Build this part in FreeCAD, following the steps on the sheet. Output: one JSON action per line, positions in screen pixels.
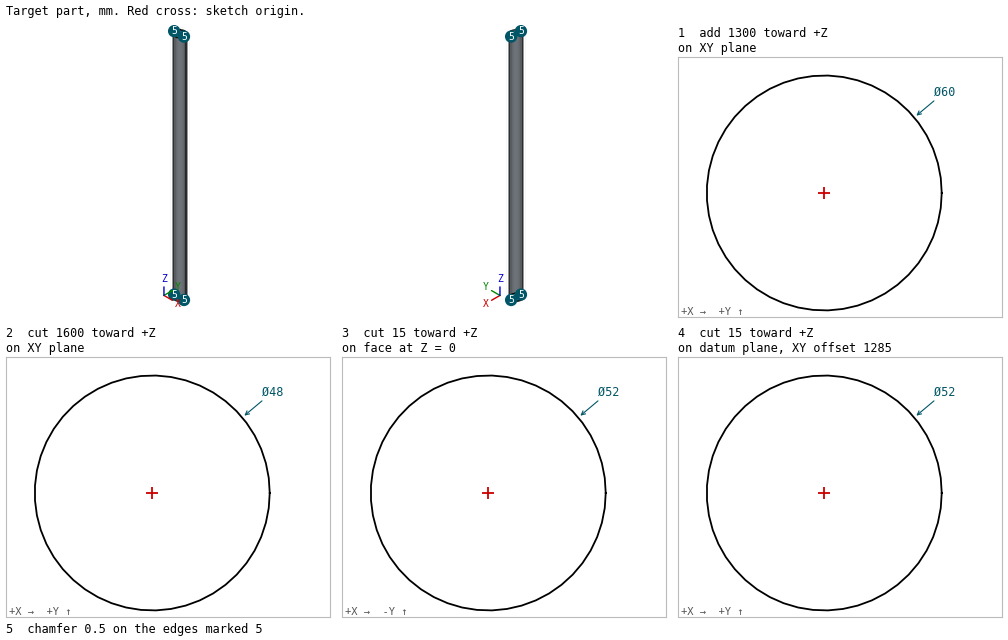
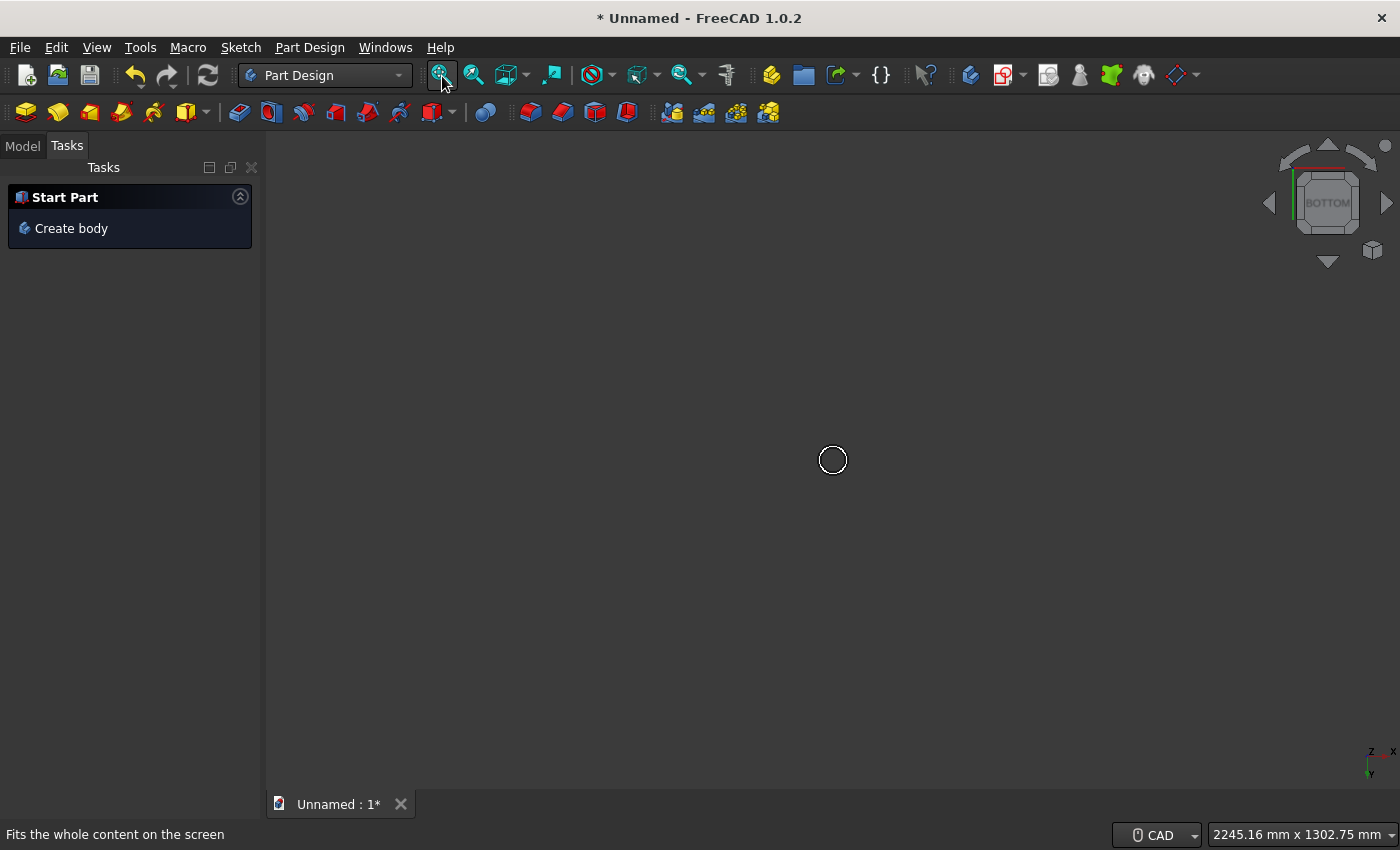
{"action": "scroll", "coordinate": [837, 472], "scroll_direction": "up", "scroll_amount": 11}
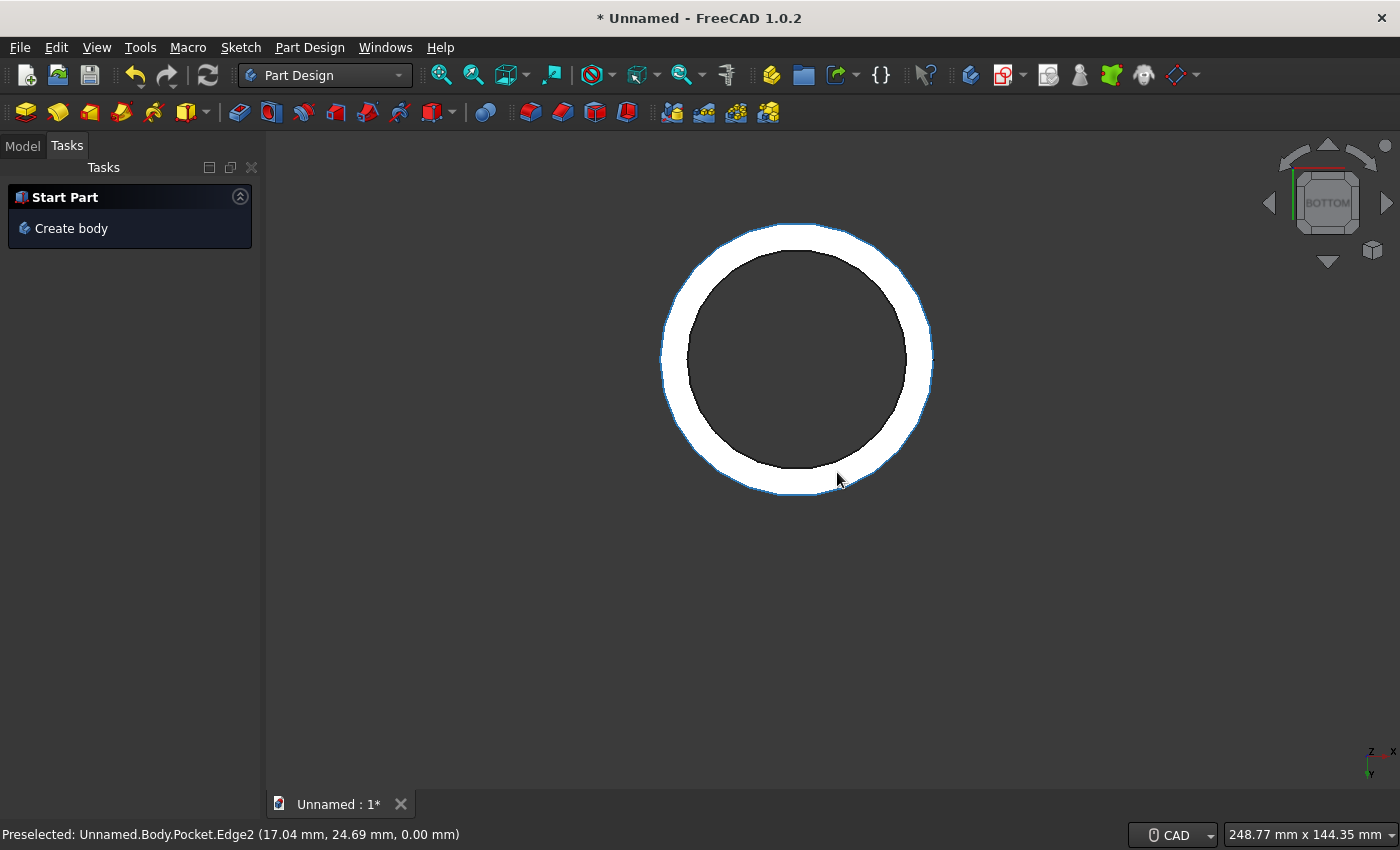
{"action": "left_click", "coordinate": [836, 476]}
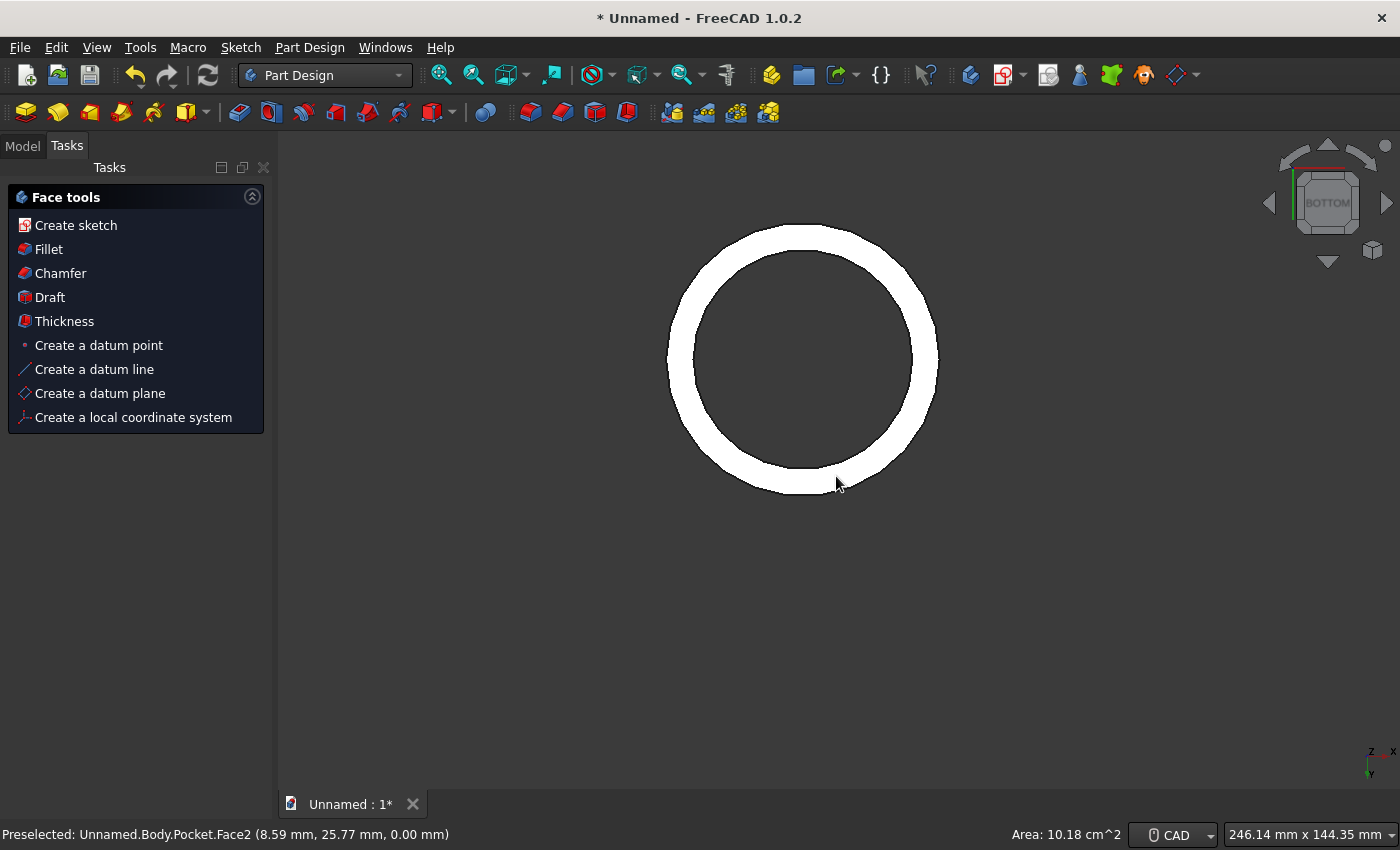
{"action": "left_click", "coordinate": [1004, 76]}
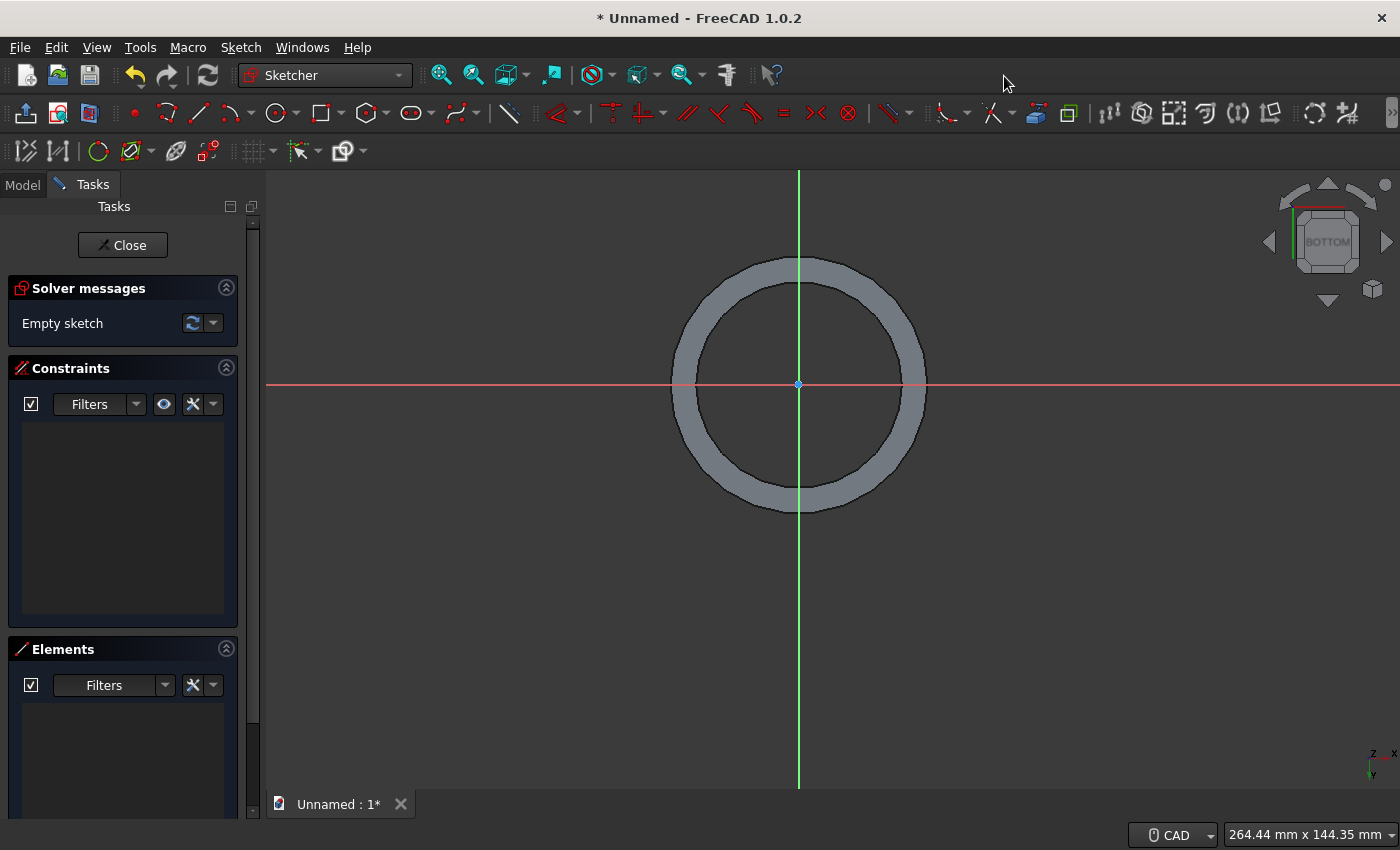
{"action": "scroll", "coordinate": [841, 270], "scroll_direction": "up", "scroll_amount": 3}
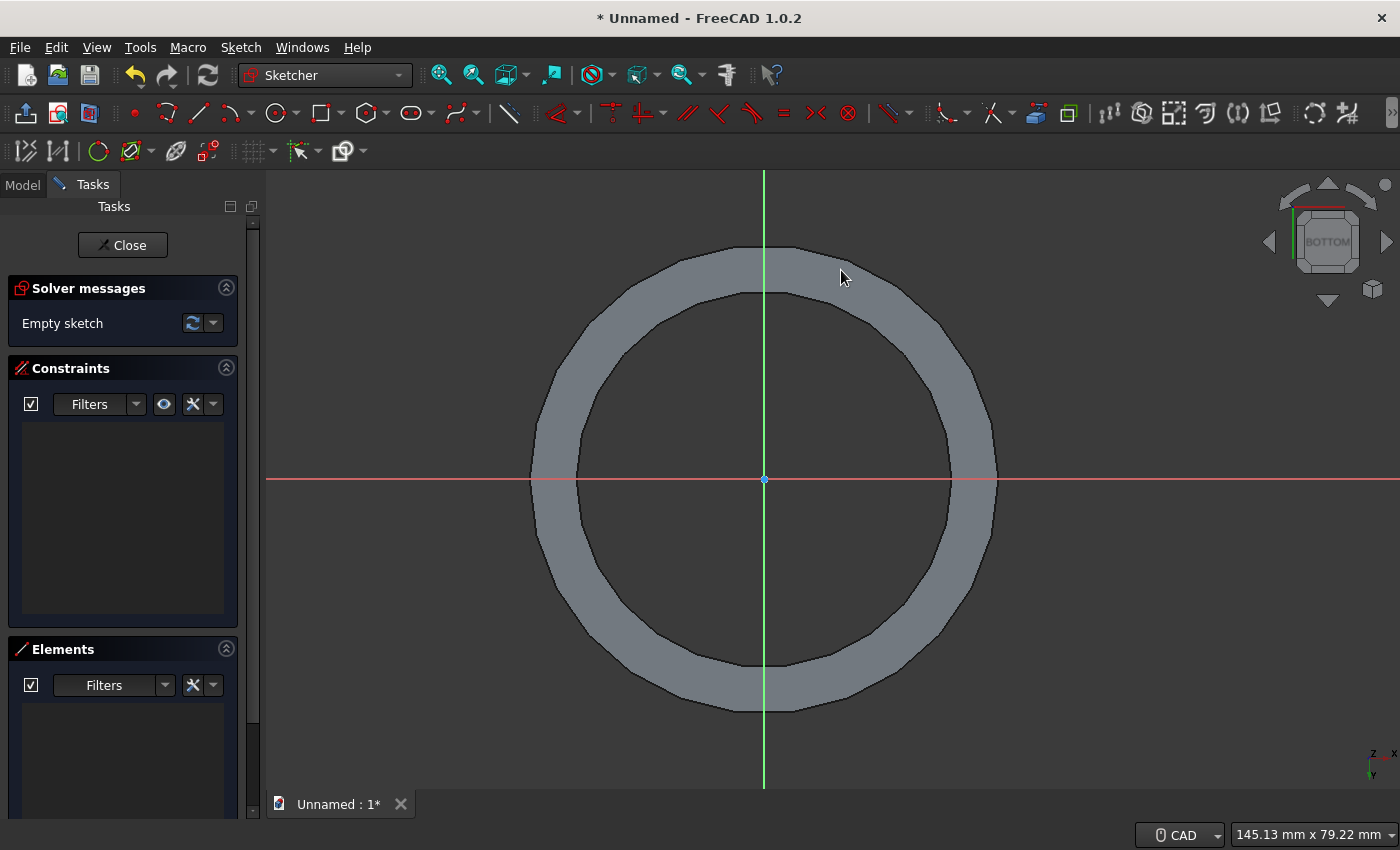
{"action": "left_click", "coordinate": [276, 114]}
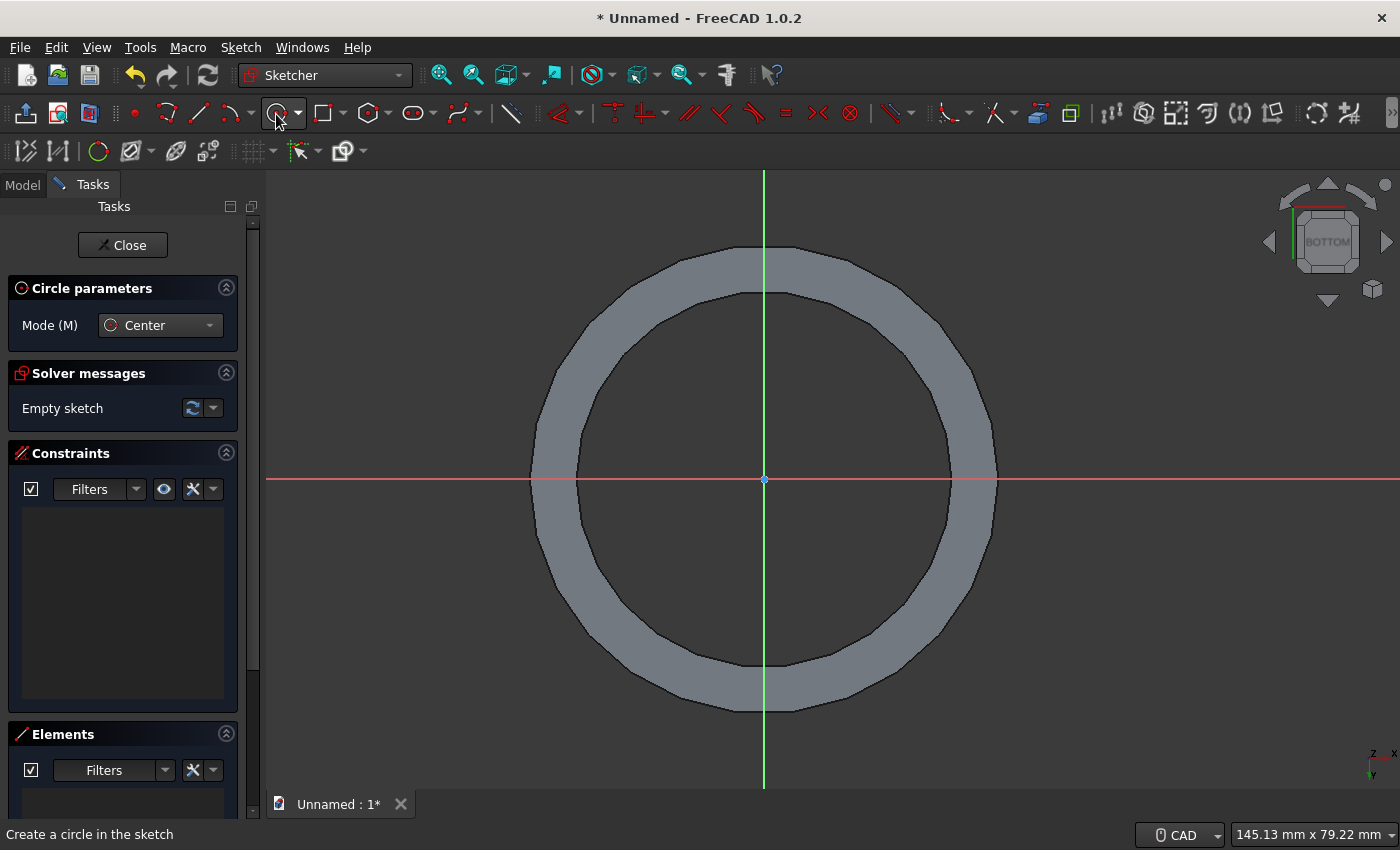
{"action": "left_click", "coordinate": [764, 479]}
{"action": "mouse_move", "coordinate": [908, 336]}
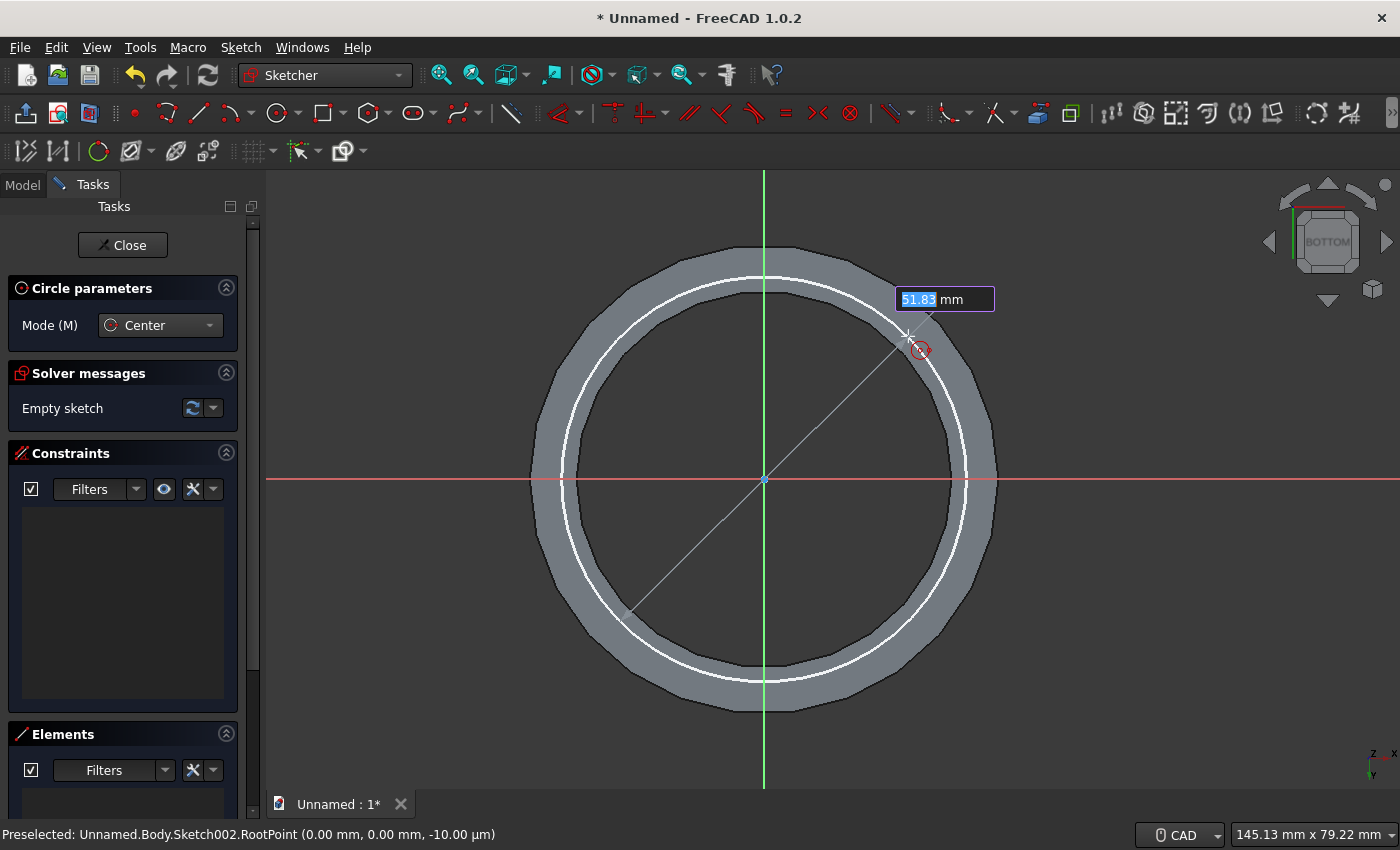
{"action": "type", "text": "52"}
{"action": "key", "text": "Return"}
{"action": "key", "text": "Escape"}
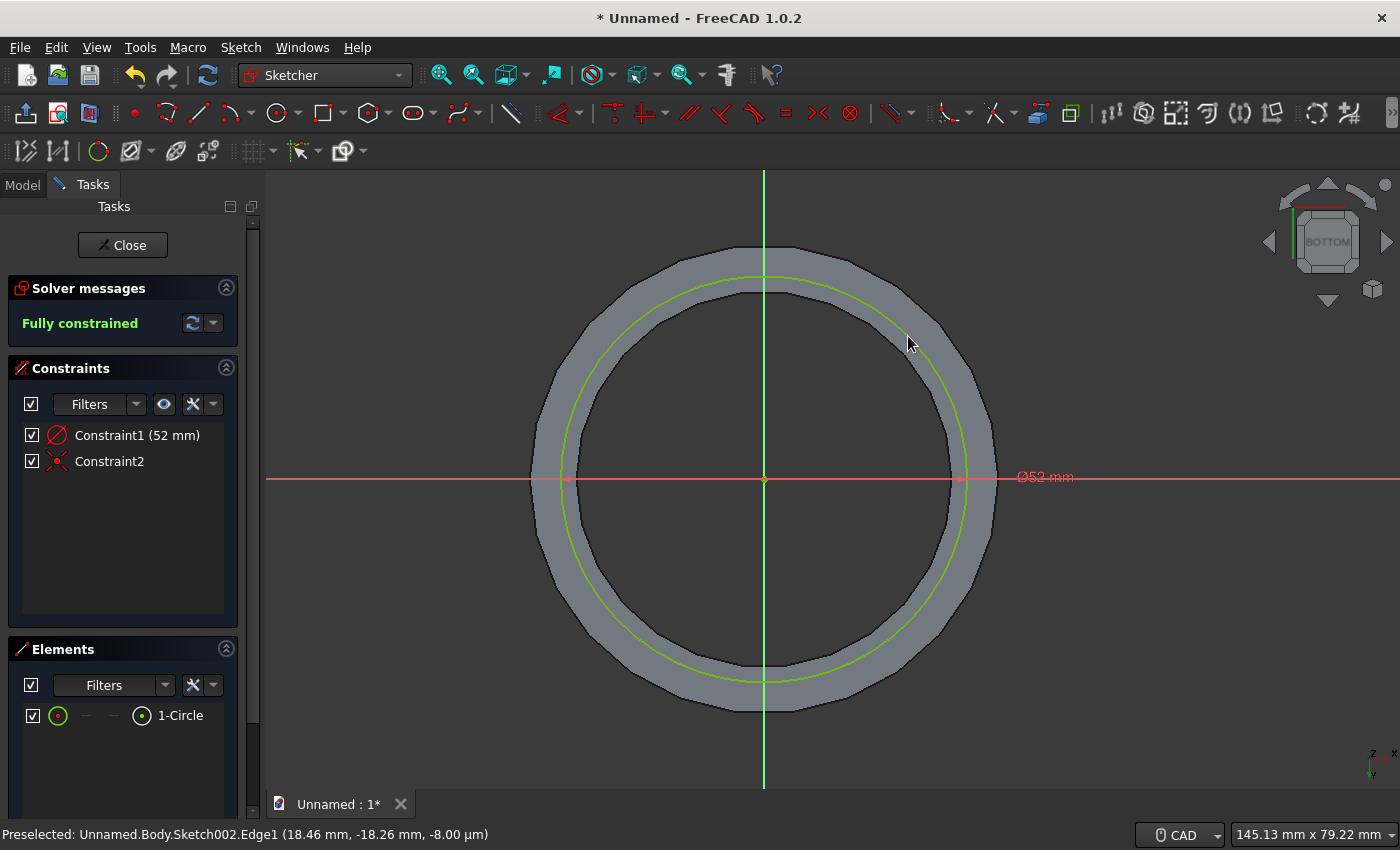
{"action": "left_click", "coordinate": [123, 245]}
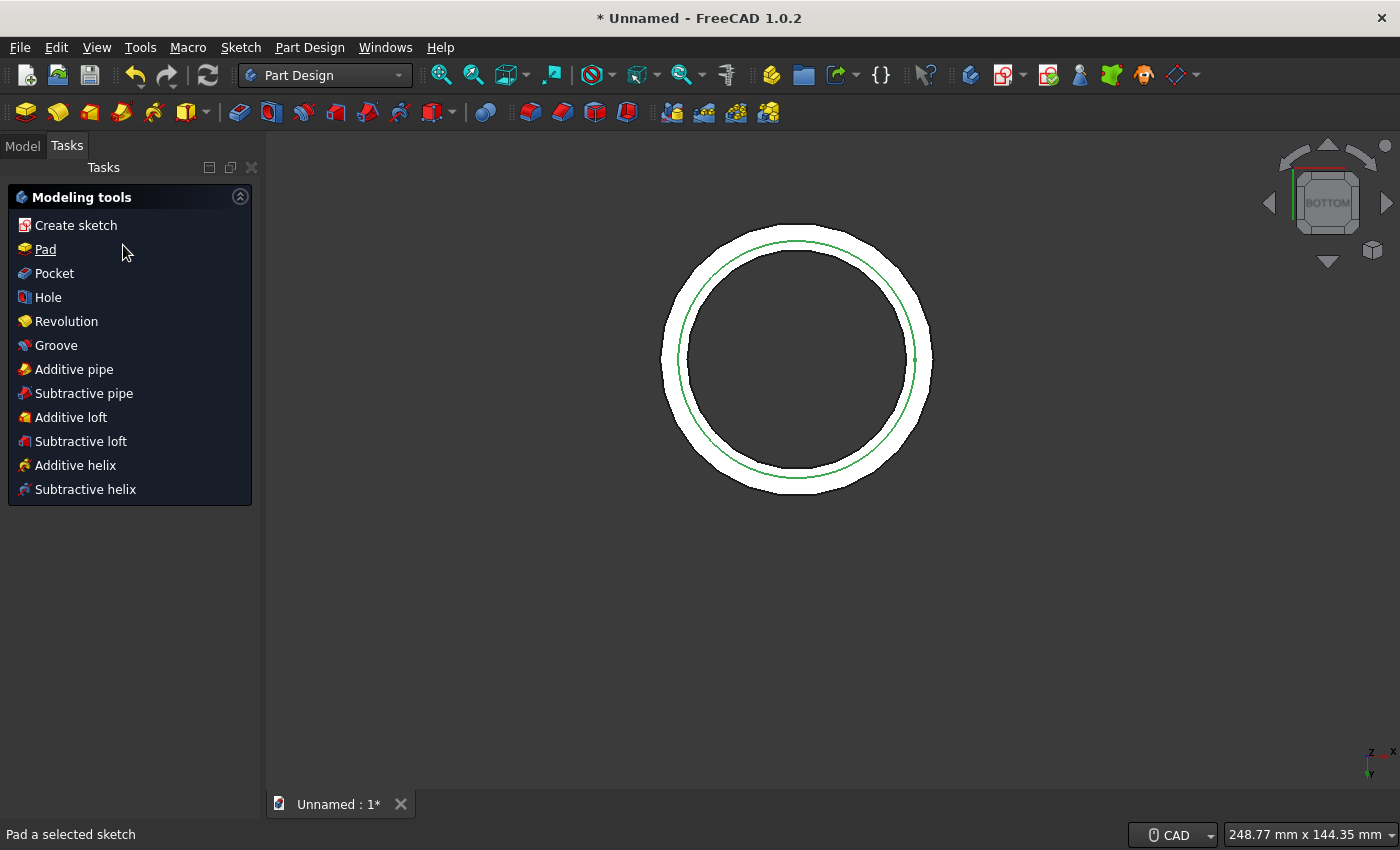
{"action": "left_click", "coordinate": [240, 112]}